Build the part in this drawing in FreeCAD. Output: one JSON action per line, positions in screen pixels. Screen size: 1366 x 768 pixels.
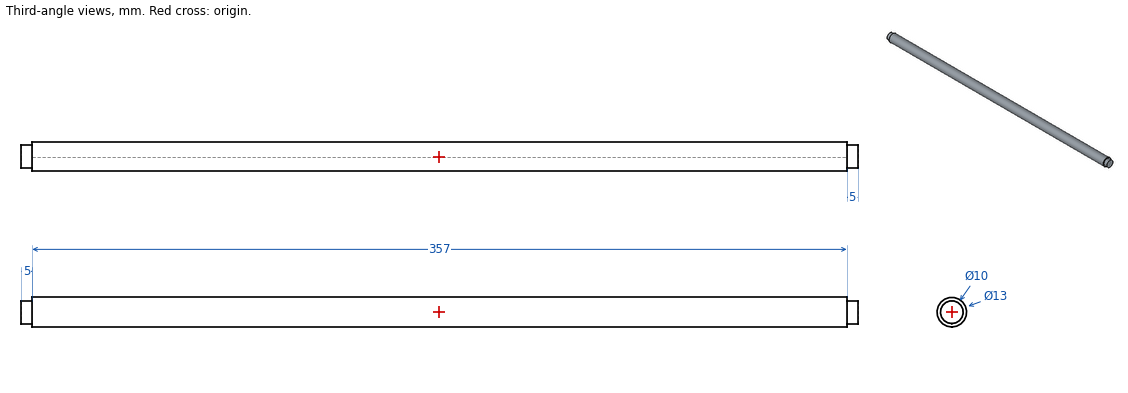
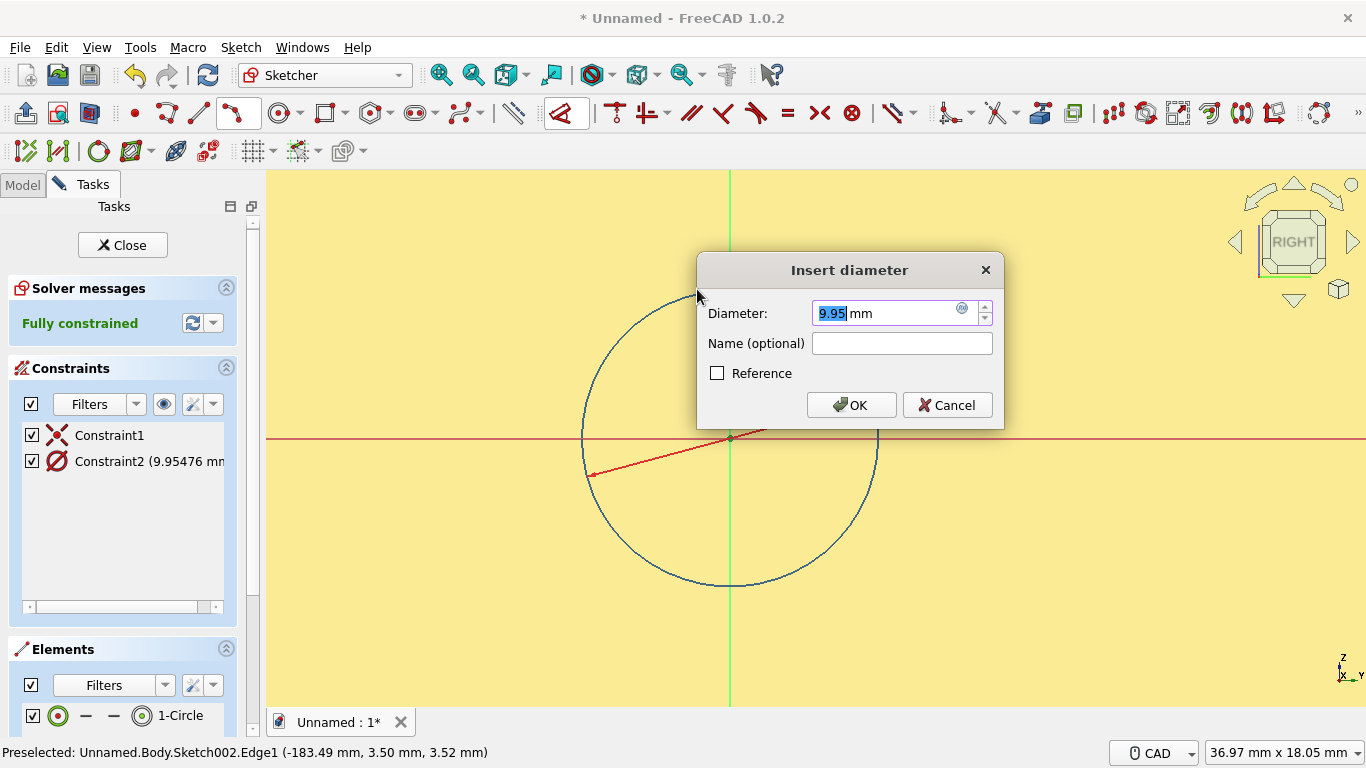
{"action": "type", "text": "10"}
{"action": "key", "text": "Return"}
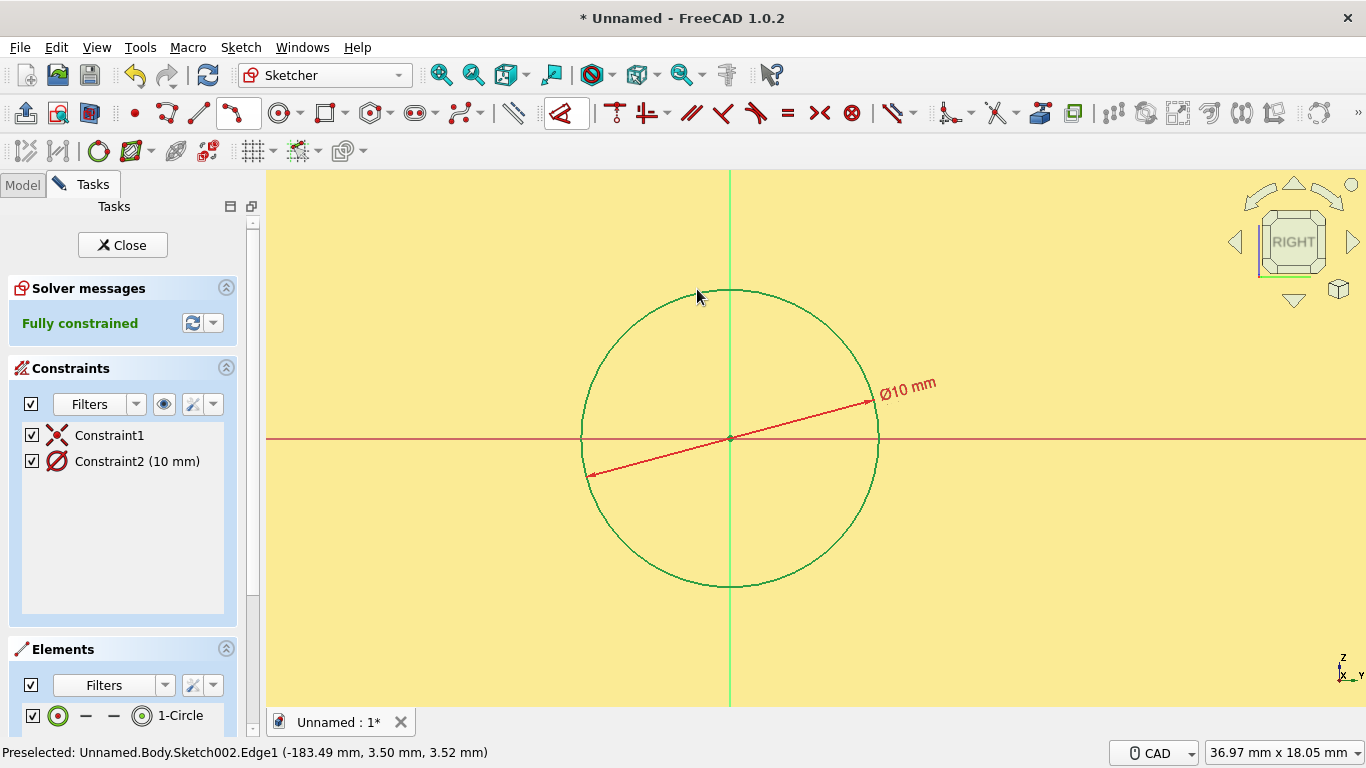
{"action": "left_click", "coordinate": [123, 245]}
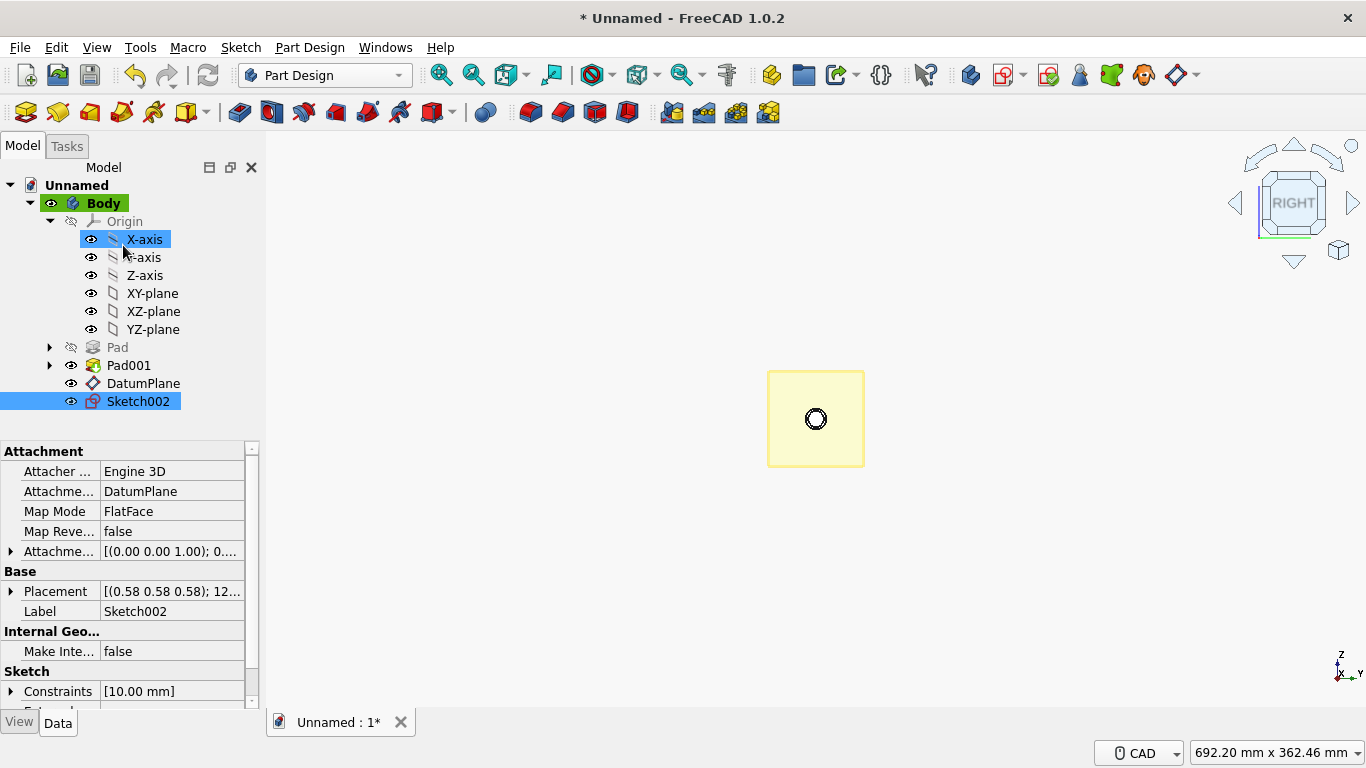
{"action": "left_click", "coordinate": [26, 112]}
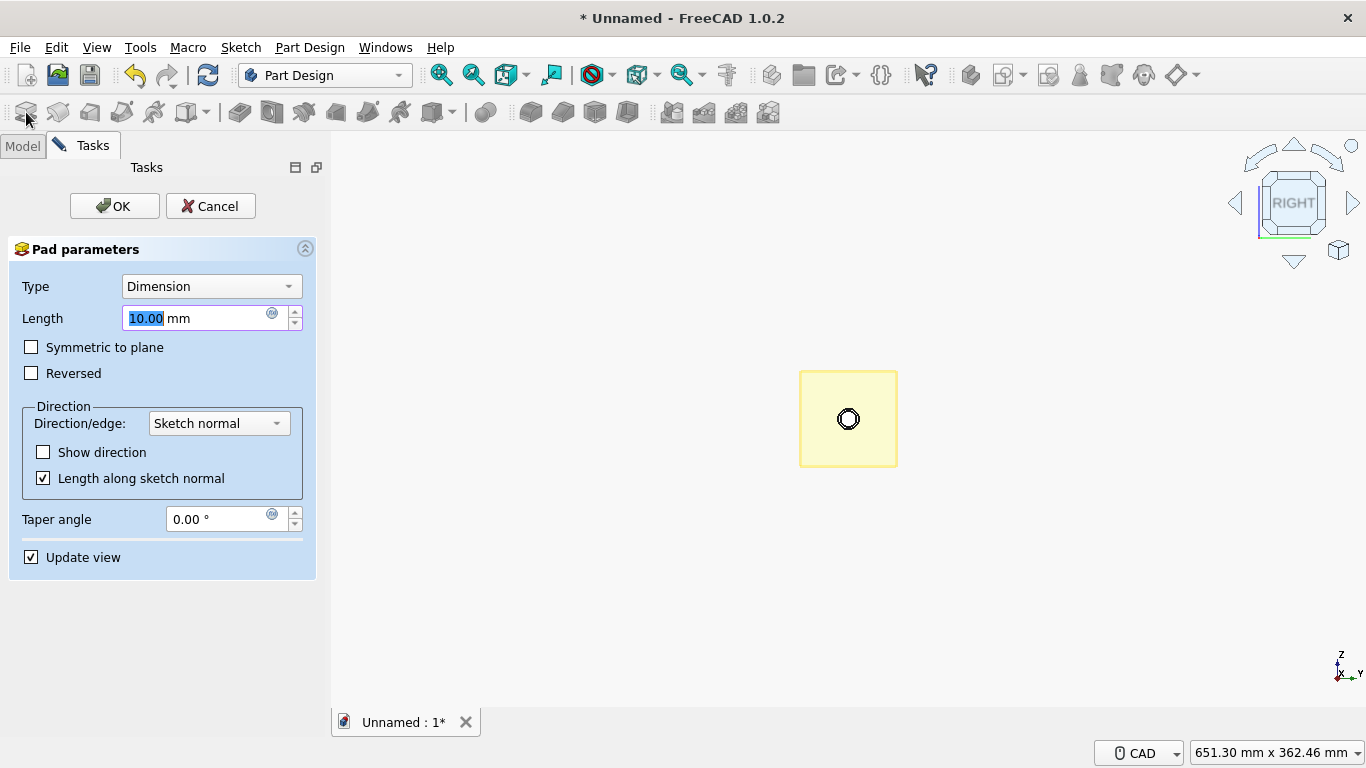
{"action": "type", "text": "5"}
{"action": "key", "text": "Tab"}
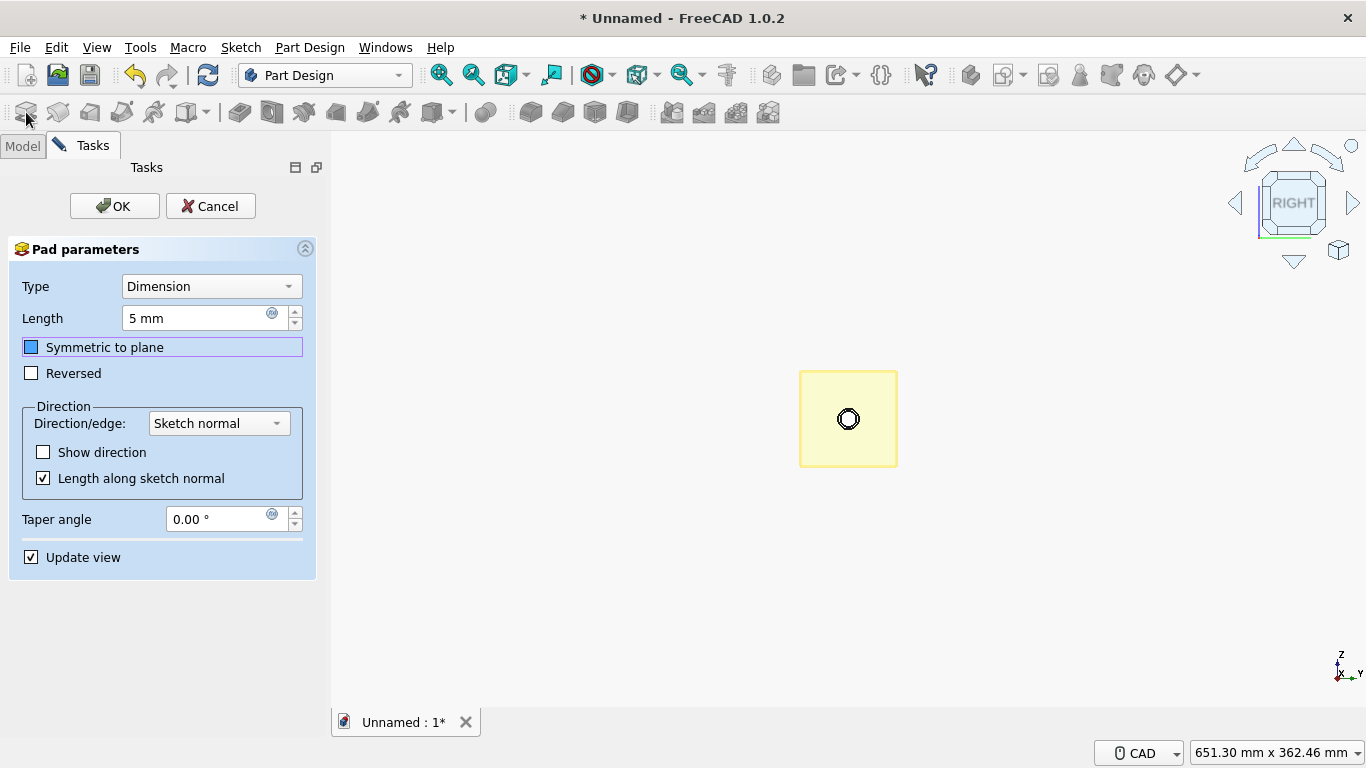
{"action": "left_click", "coordinate": [115, 206]}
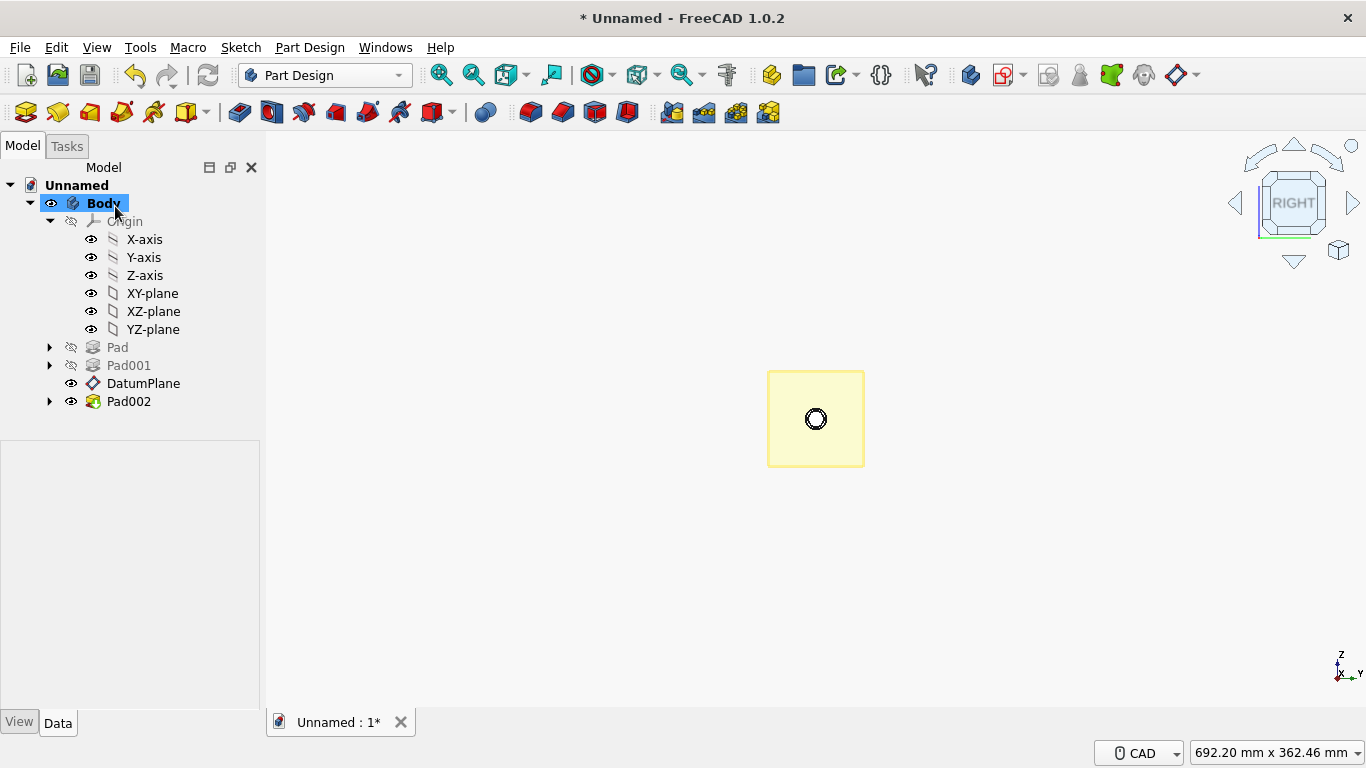
{"action": "left_click", "coordinate": [116, 383]}
{"action": "key", "text": "space"}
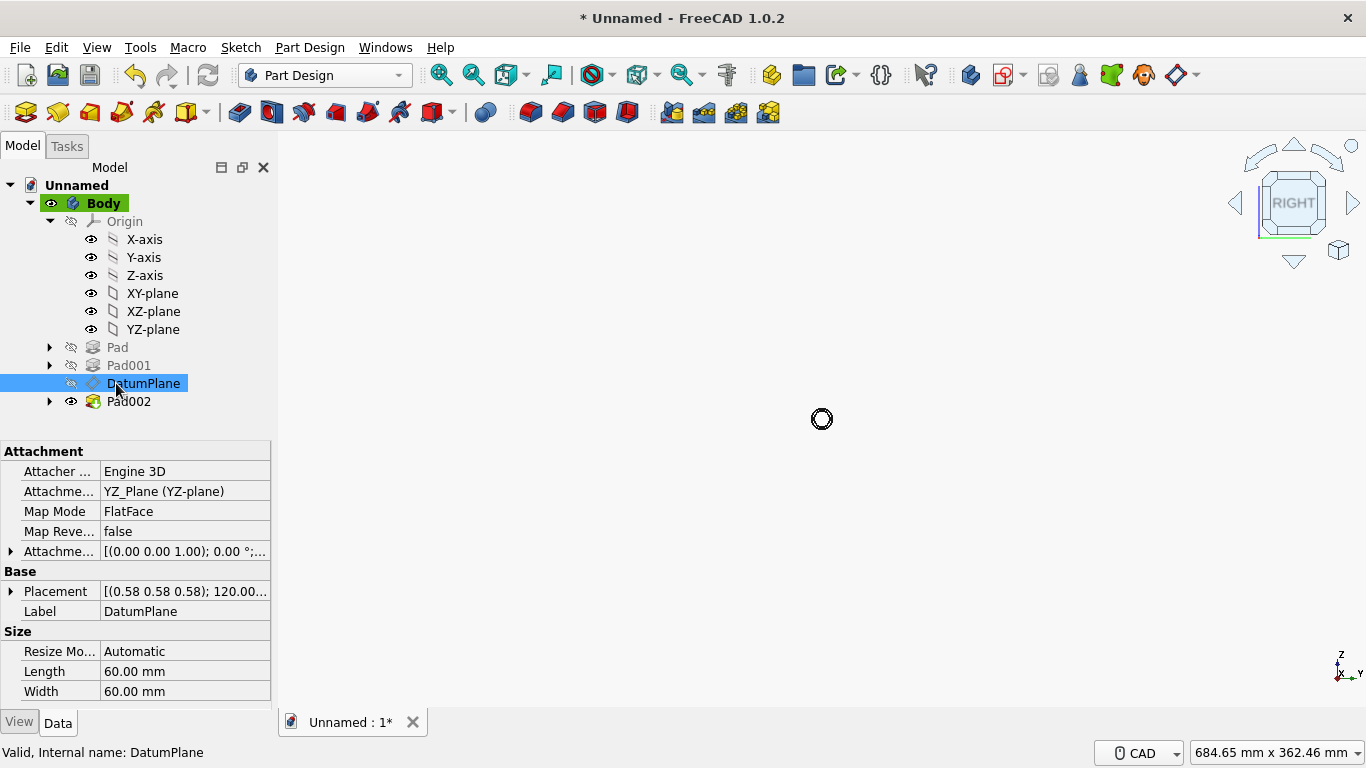
{"action": "key", "text": "0"}